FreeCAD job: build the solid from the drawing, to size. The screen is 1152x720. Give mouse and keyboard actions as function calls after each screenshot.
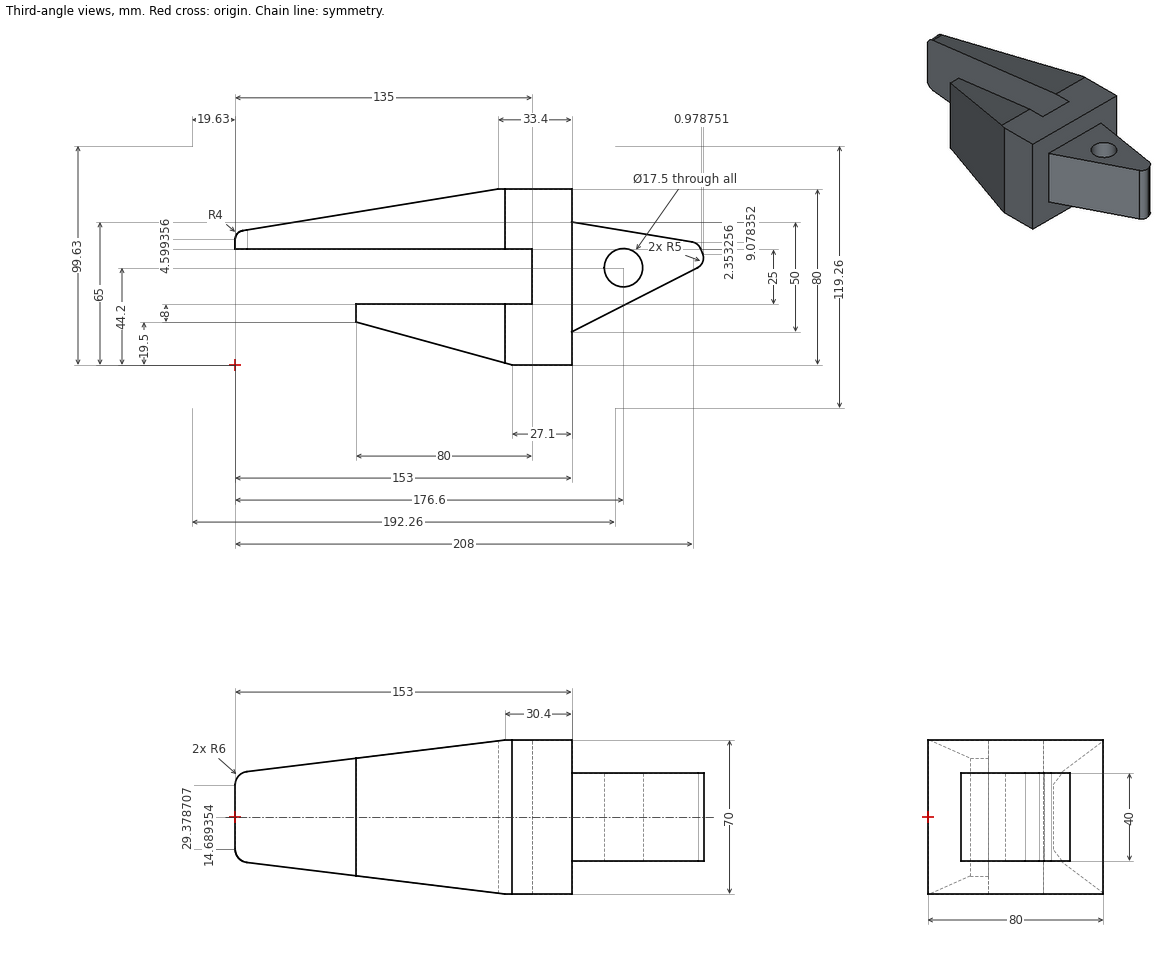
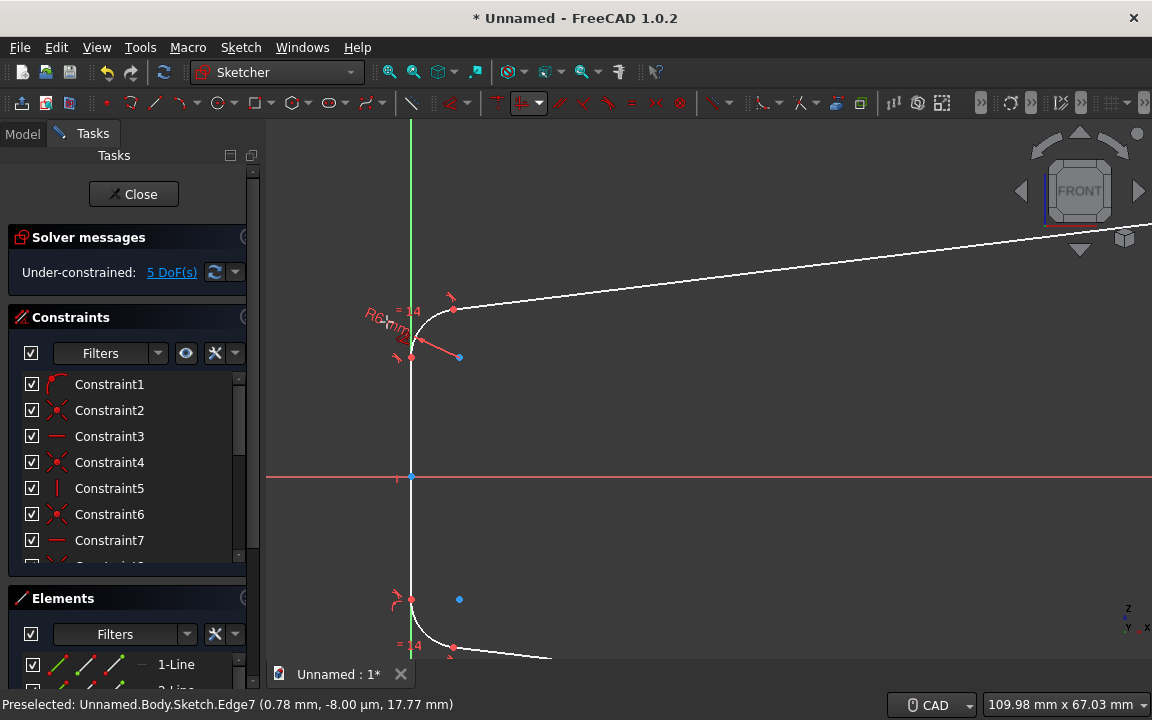
scroll(415, 338, down, 5)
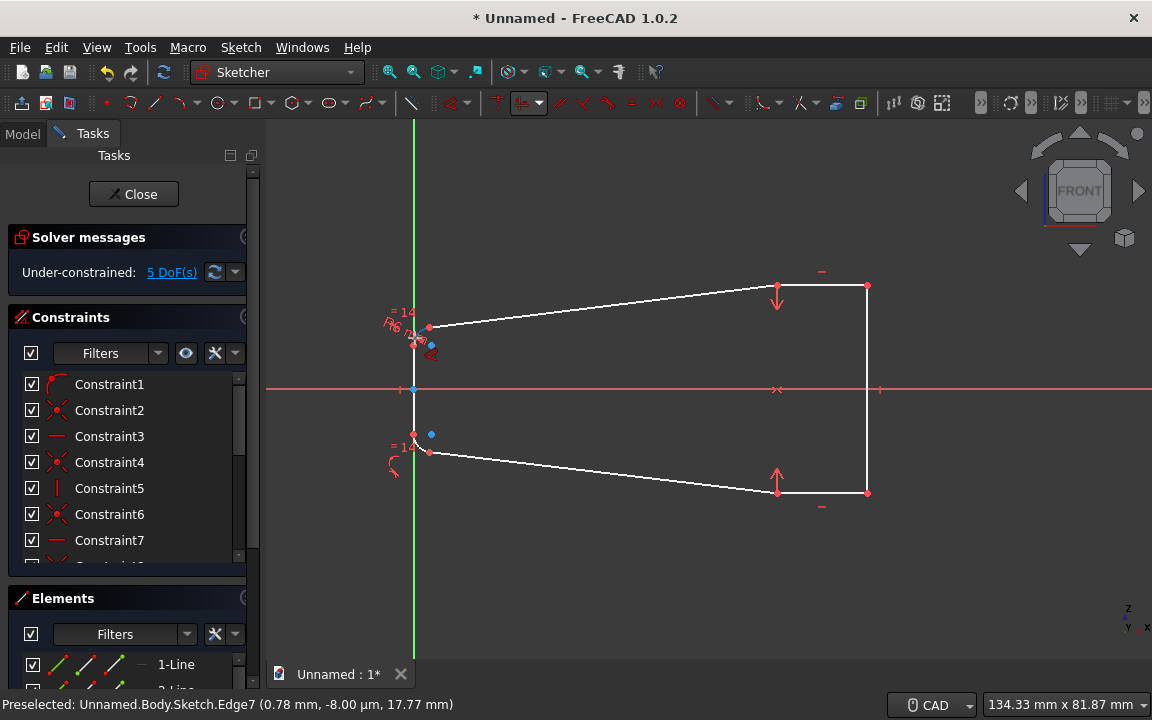
click(867, 348)
click(901, 341)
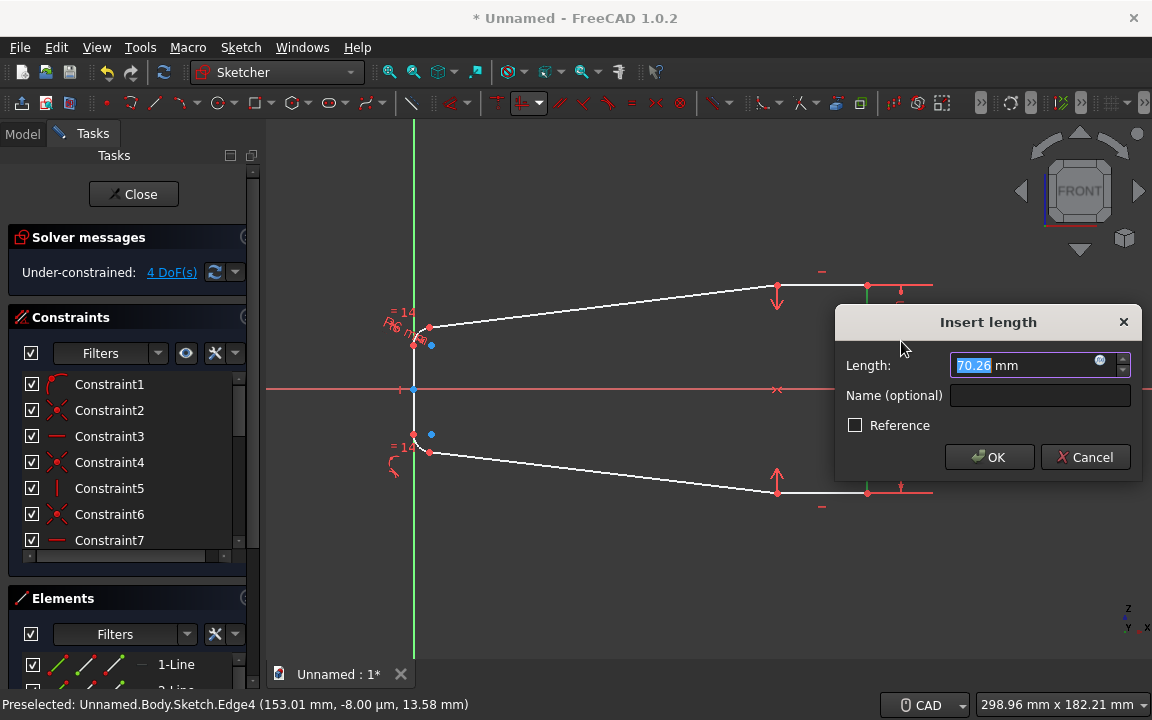
text(70)
key(Return)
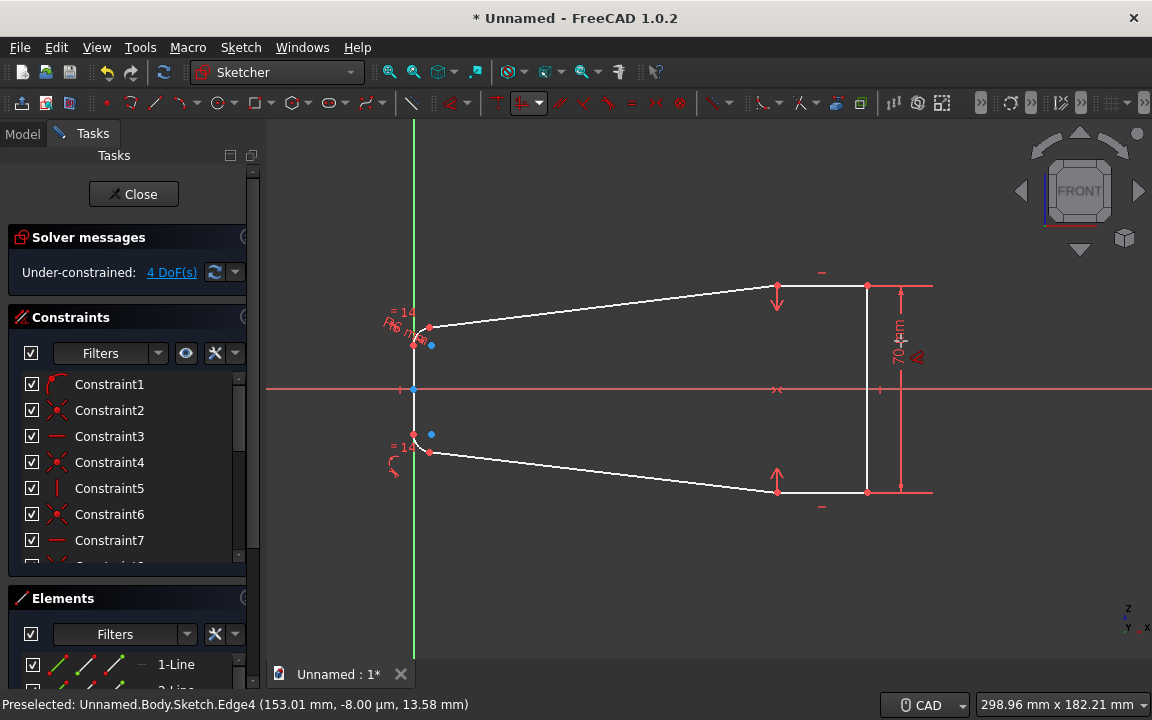
click(804, 286)
click(822, 252)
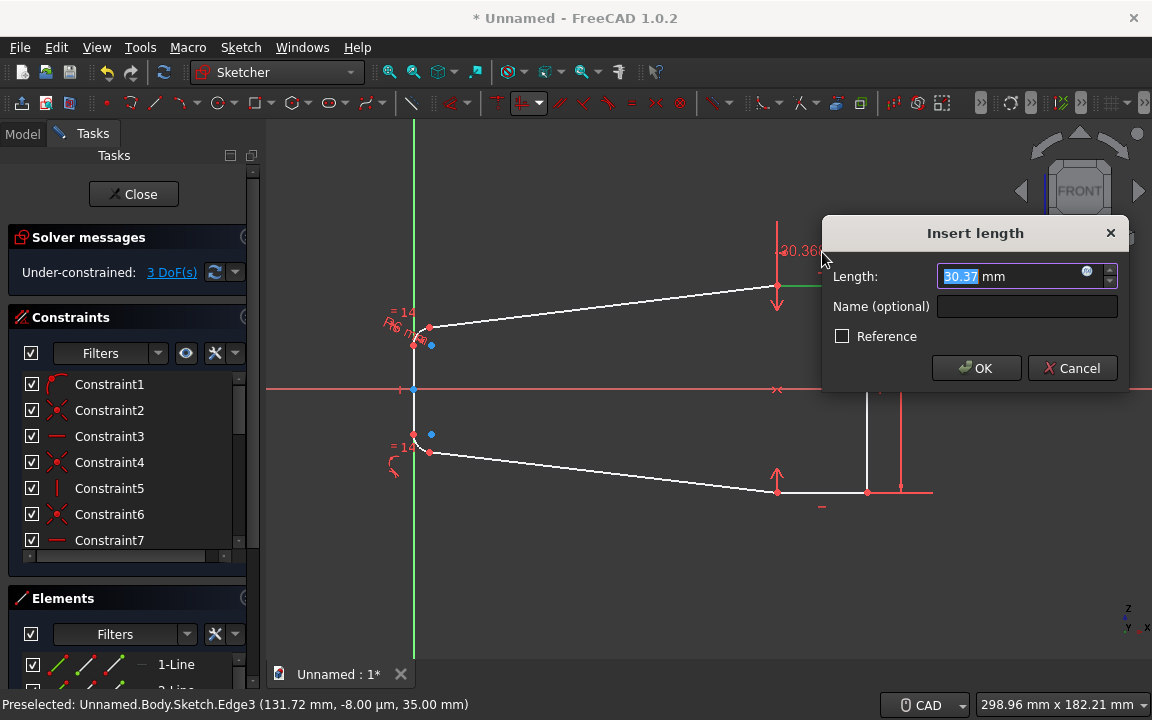
text(30.4)
key(Return)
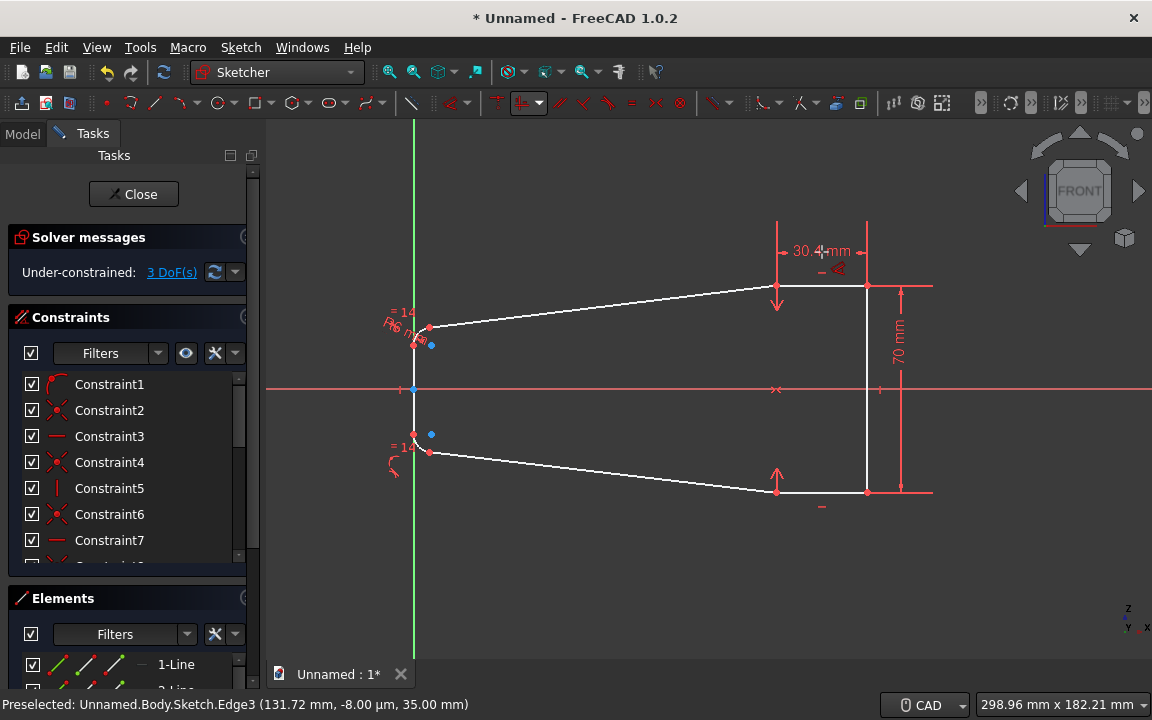
click(867, 286)
click(640, 252)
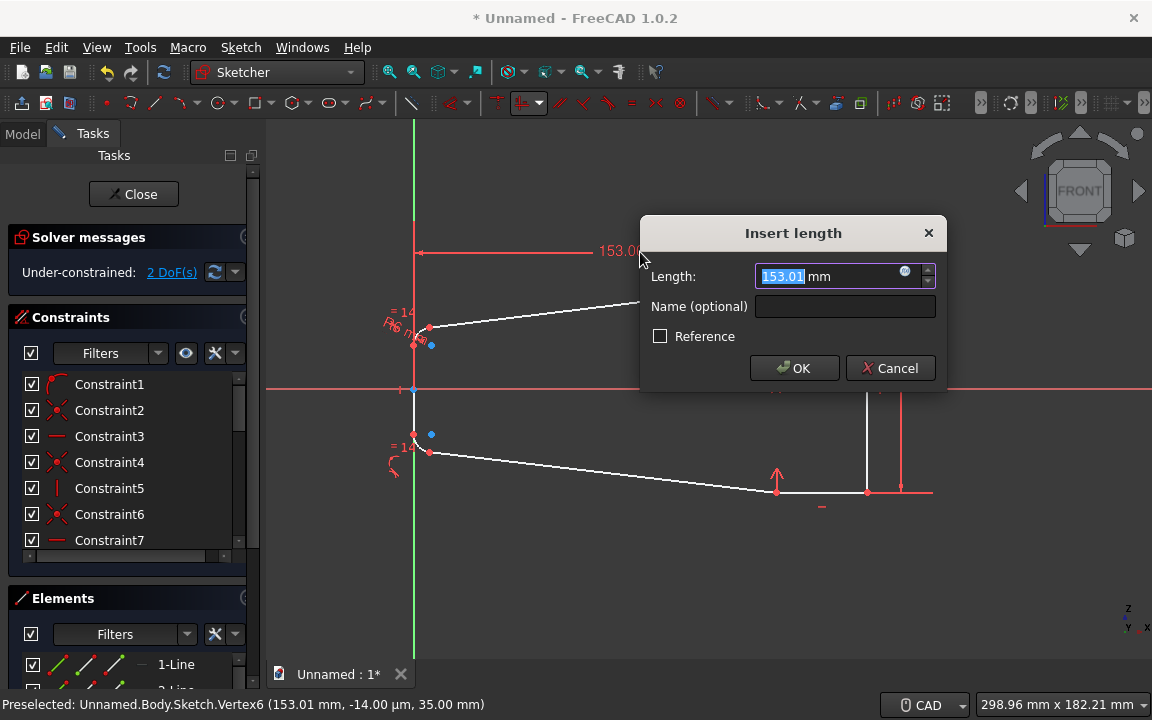
text(153)
key(Return)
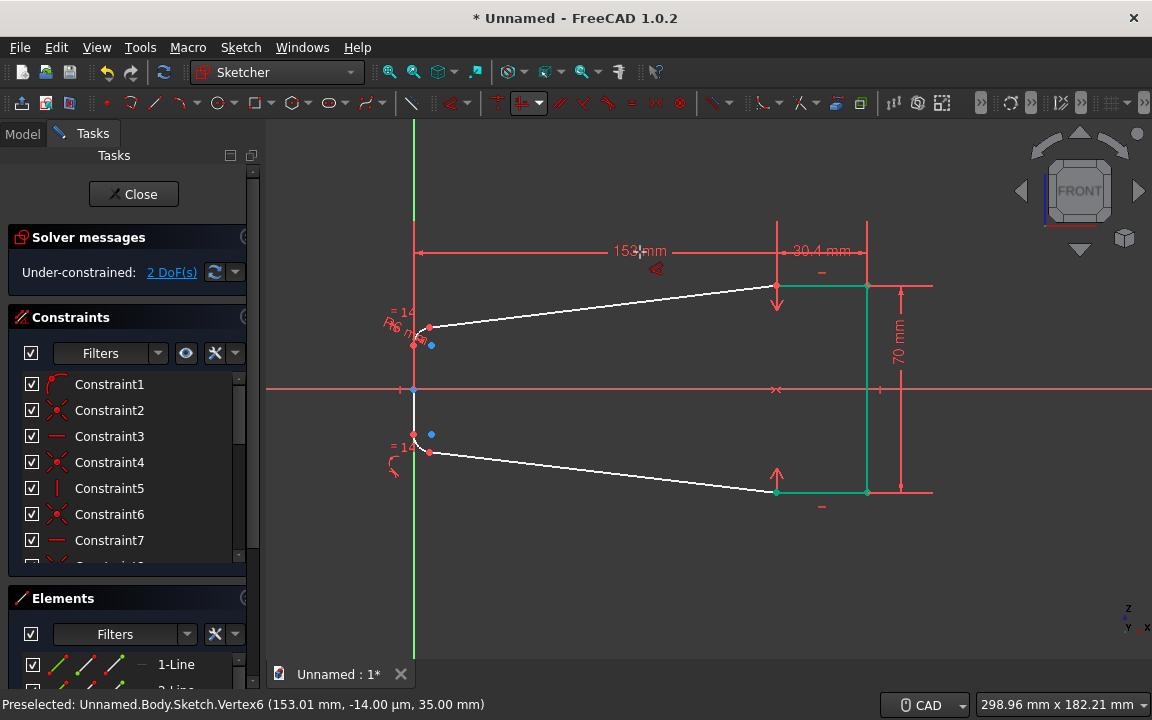
click(414, 408)
click(380, 369)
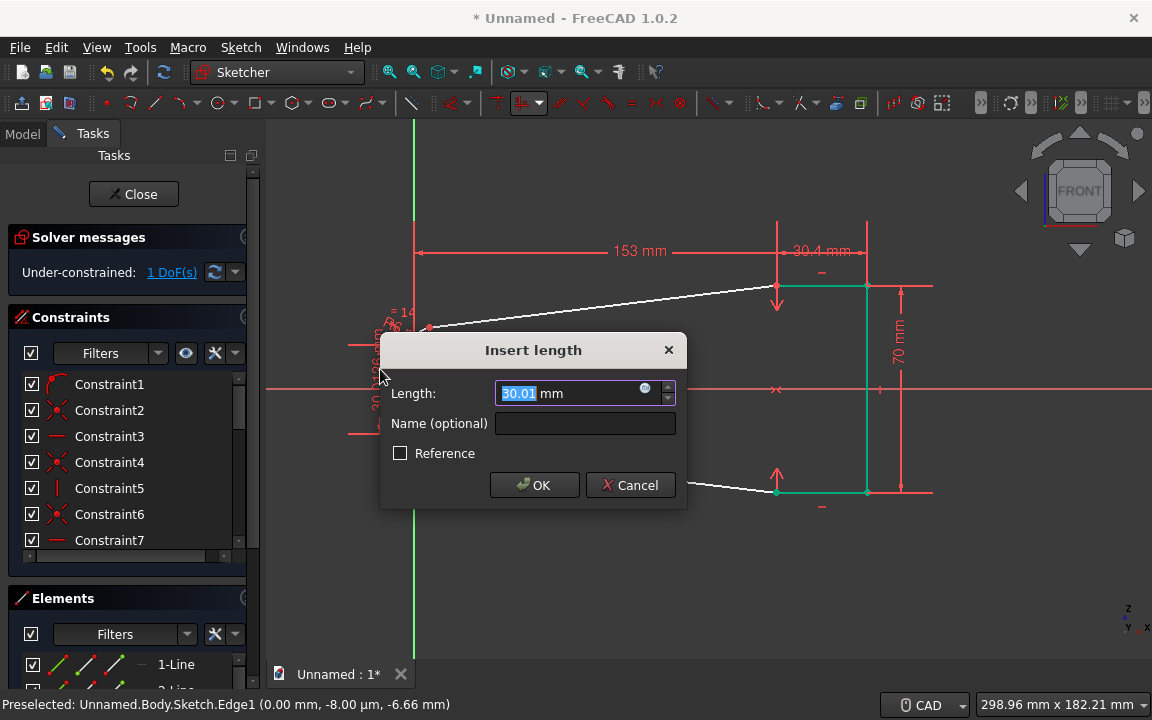
text(29.378707)
key(Return)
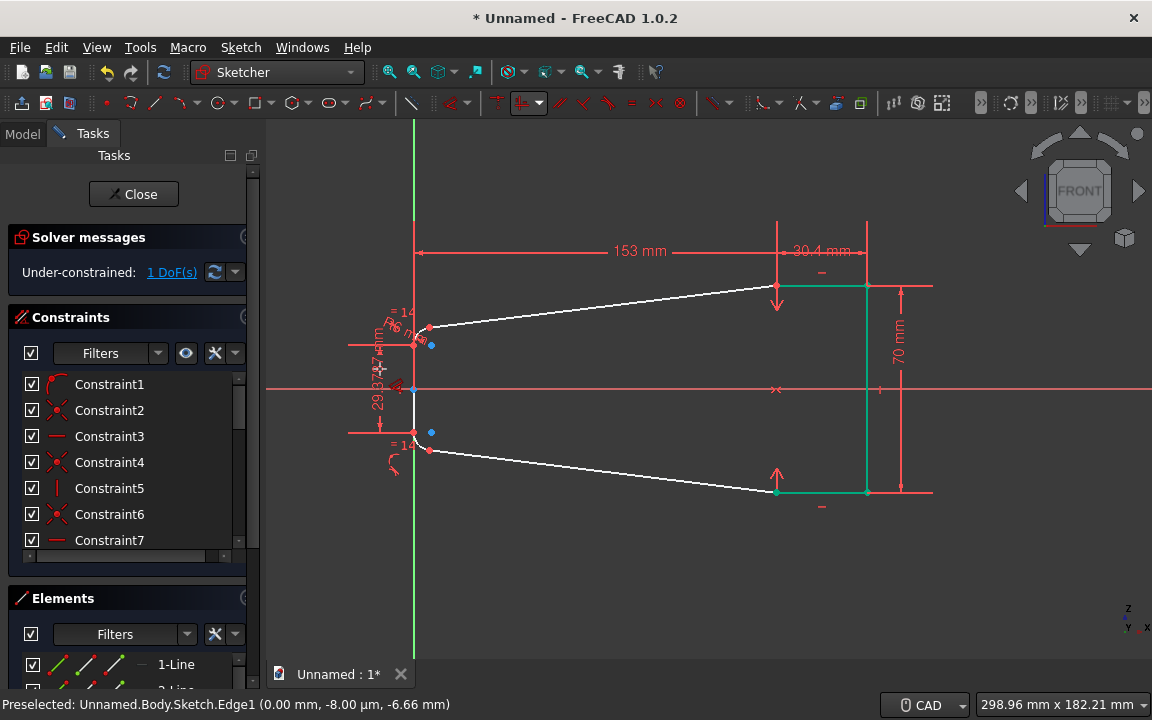
click(414, 433)
click(380, 411)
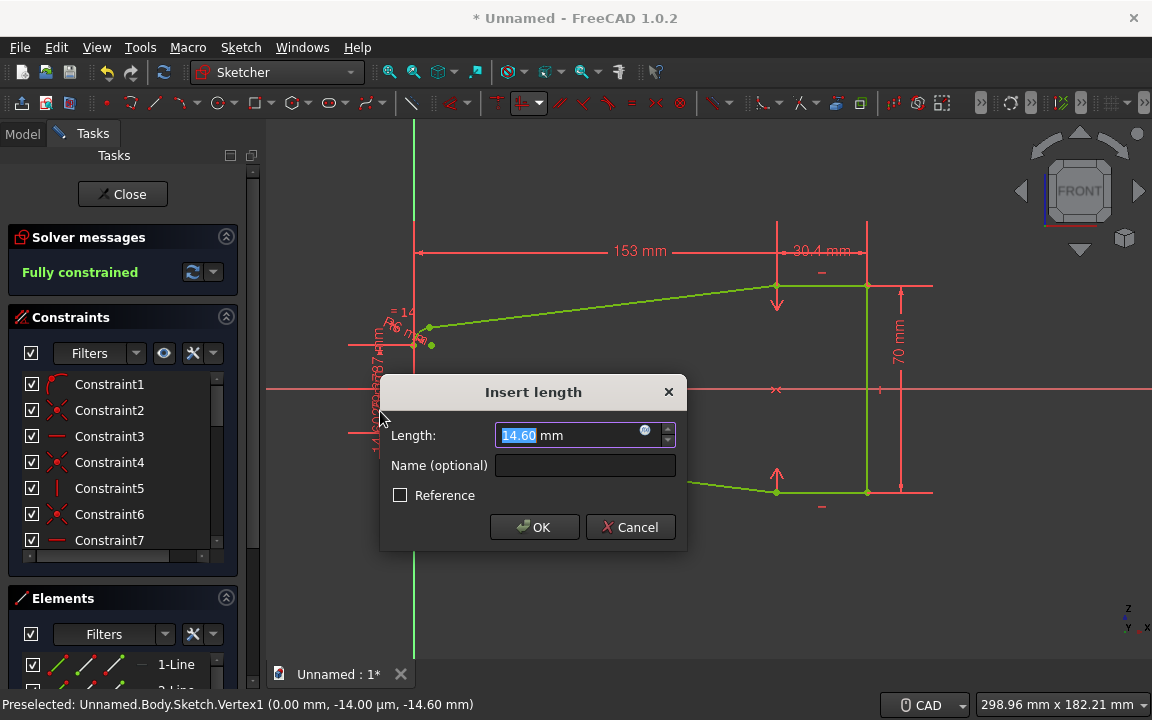
text(14.689354)
key(Return)
key(Escape)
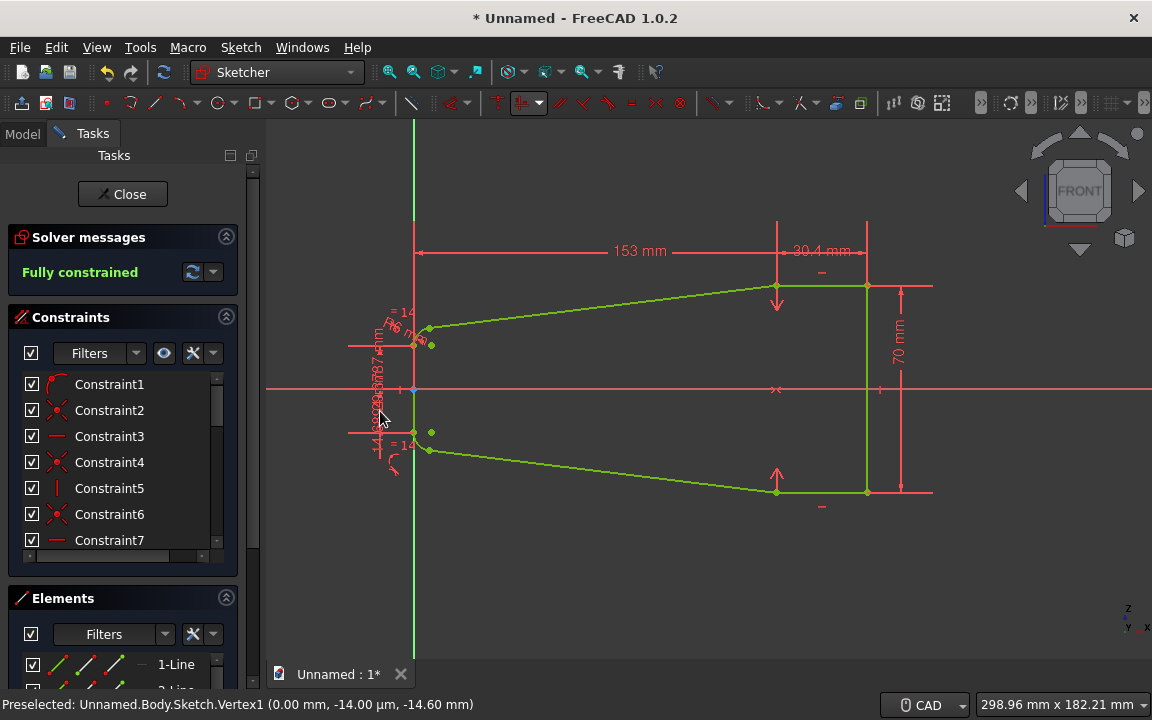
click(123, 194)